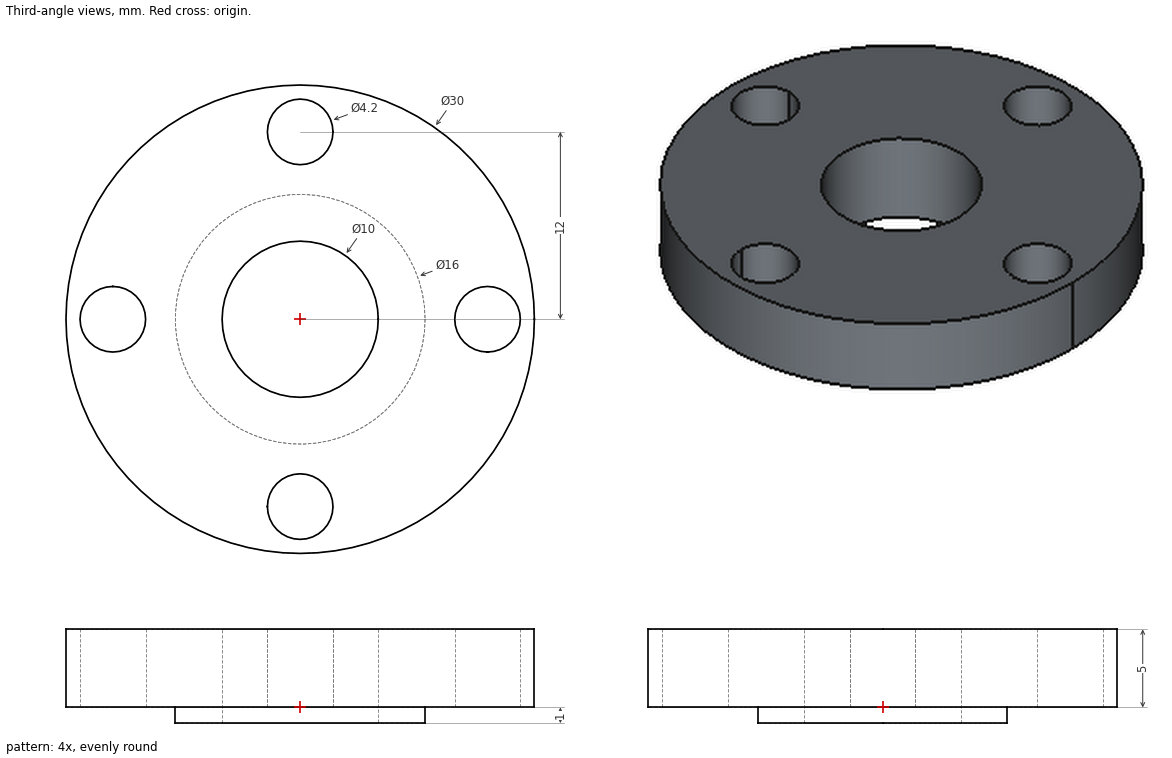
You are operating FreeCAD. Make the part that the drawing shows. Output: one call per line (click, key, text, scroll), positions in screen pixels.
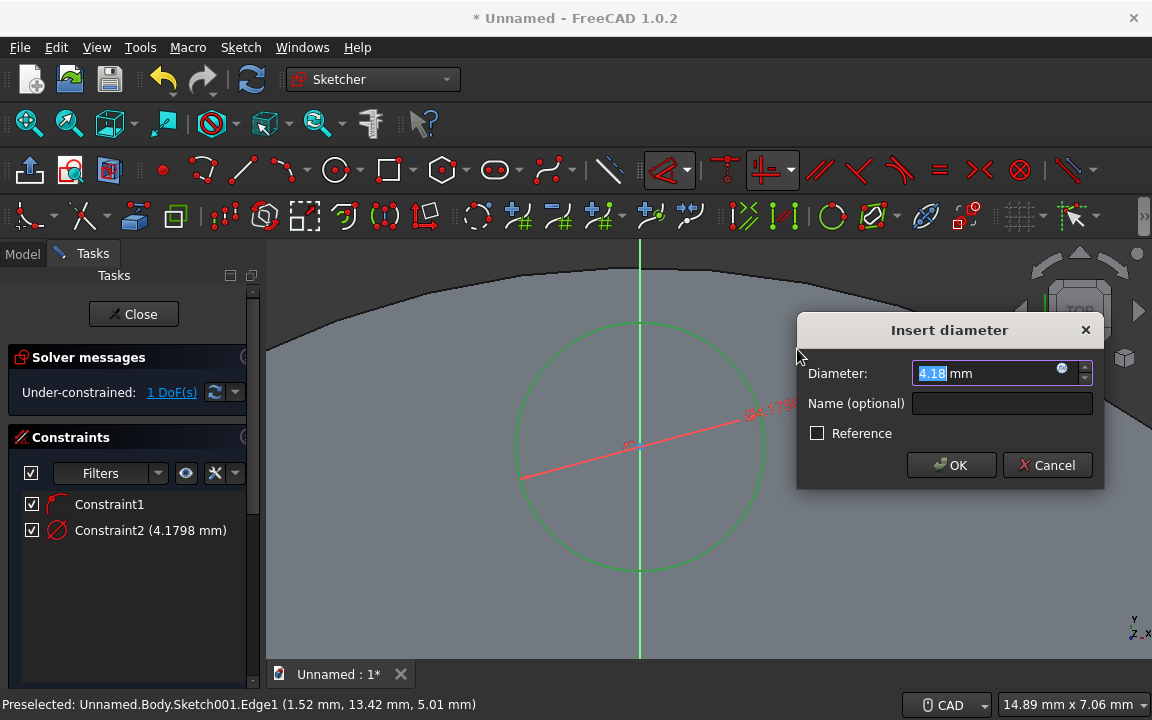
text(4.2)
key(Return)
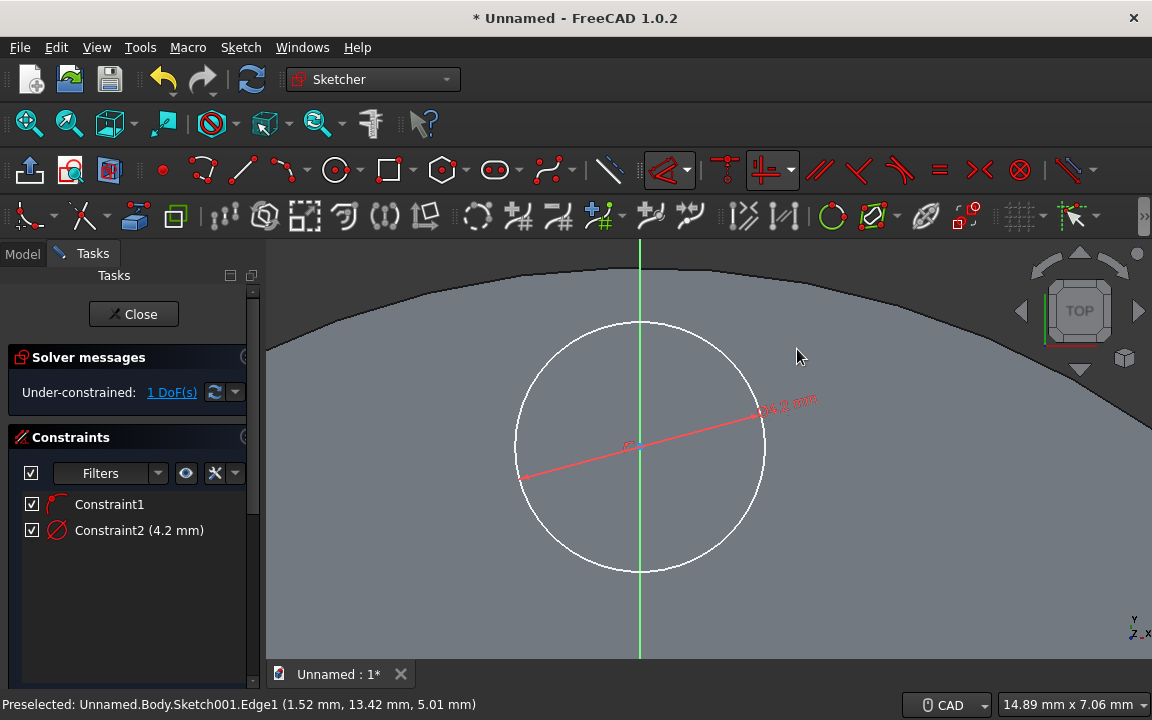
click(640, 447)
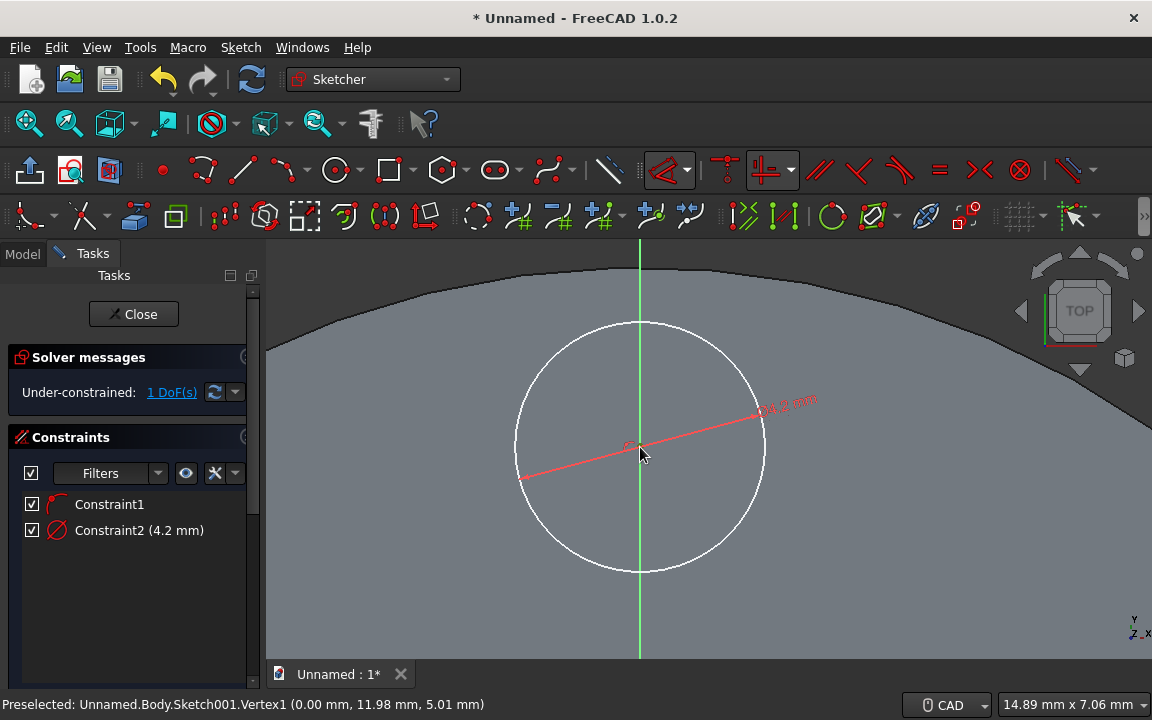
key(i)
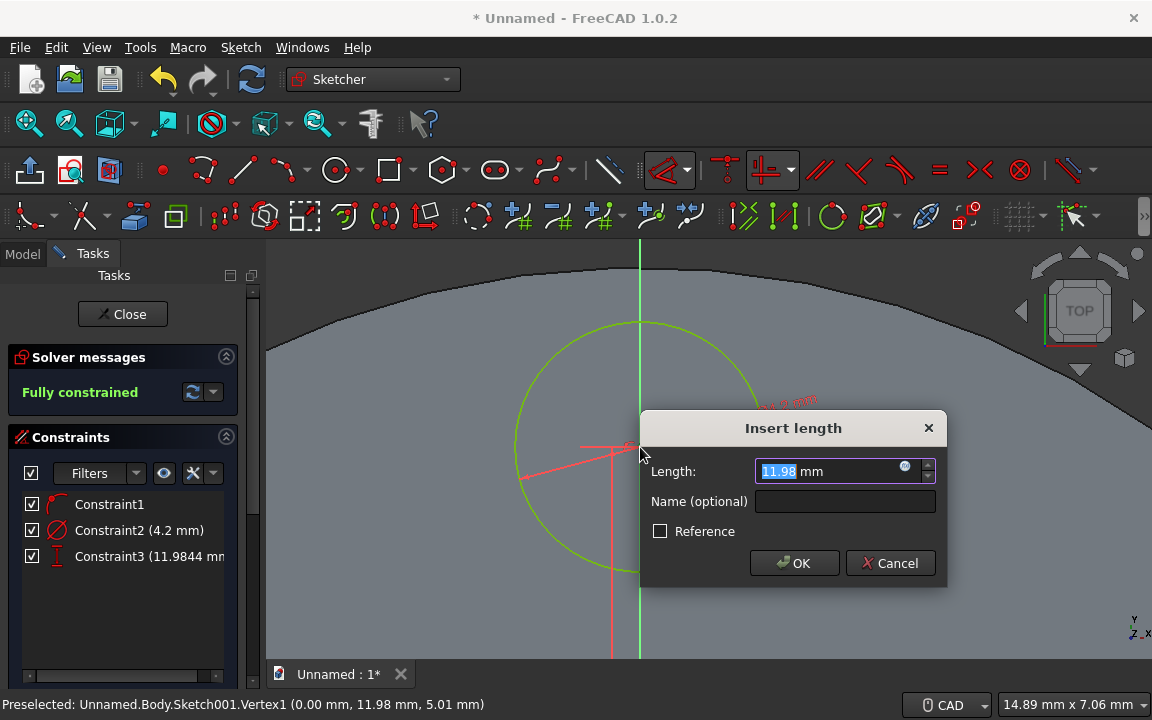
text(12)
key(Return)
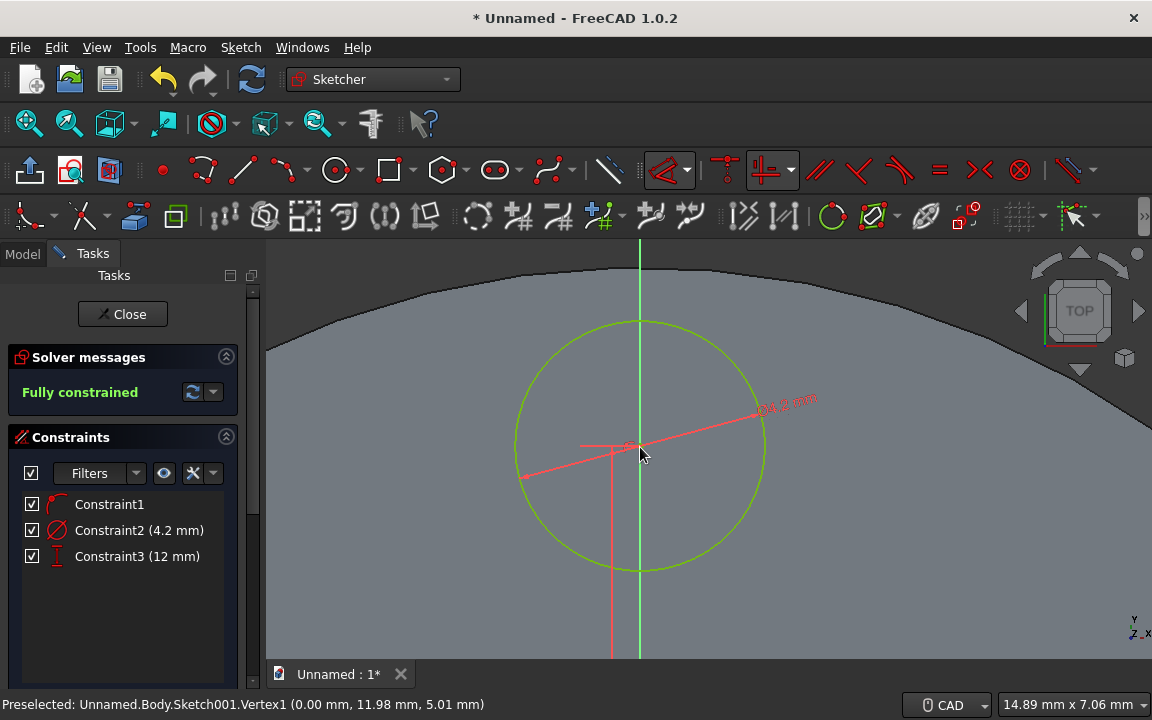
click(123, 314)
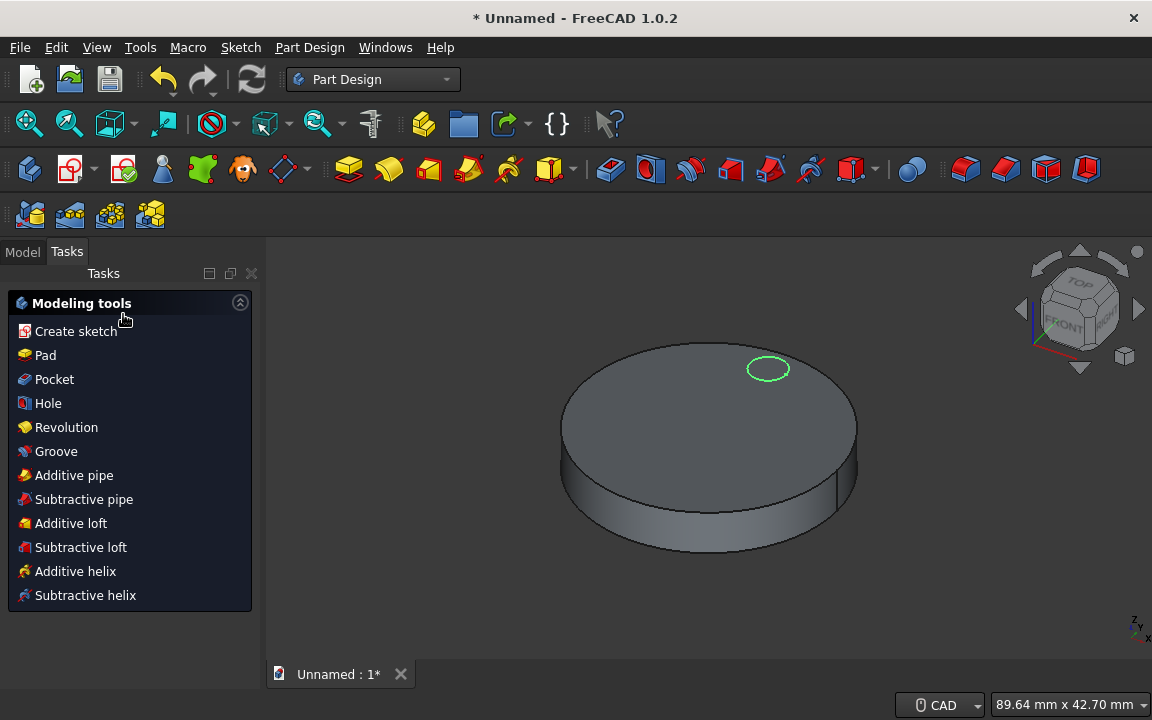
click(612, 170)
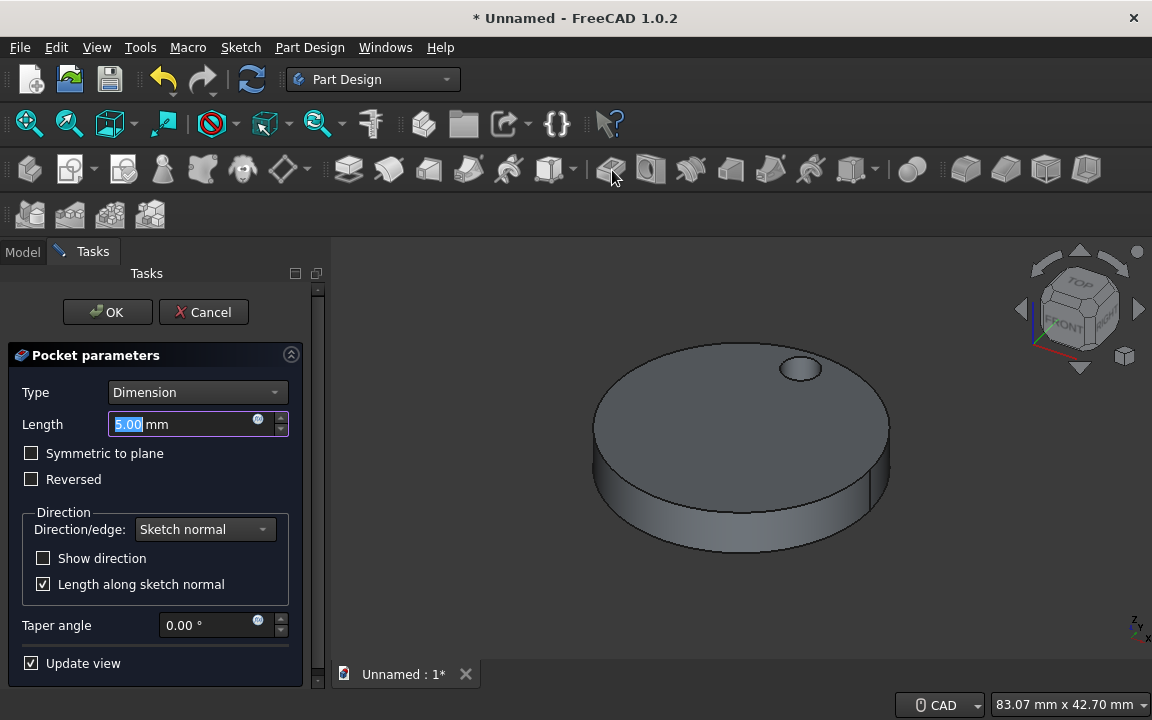
click(198, 392)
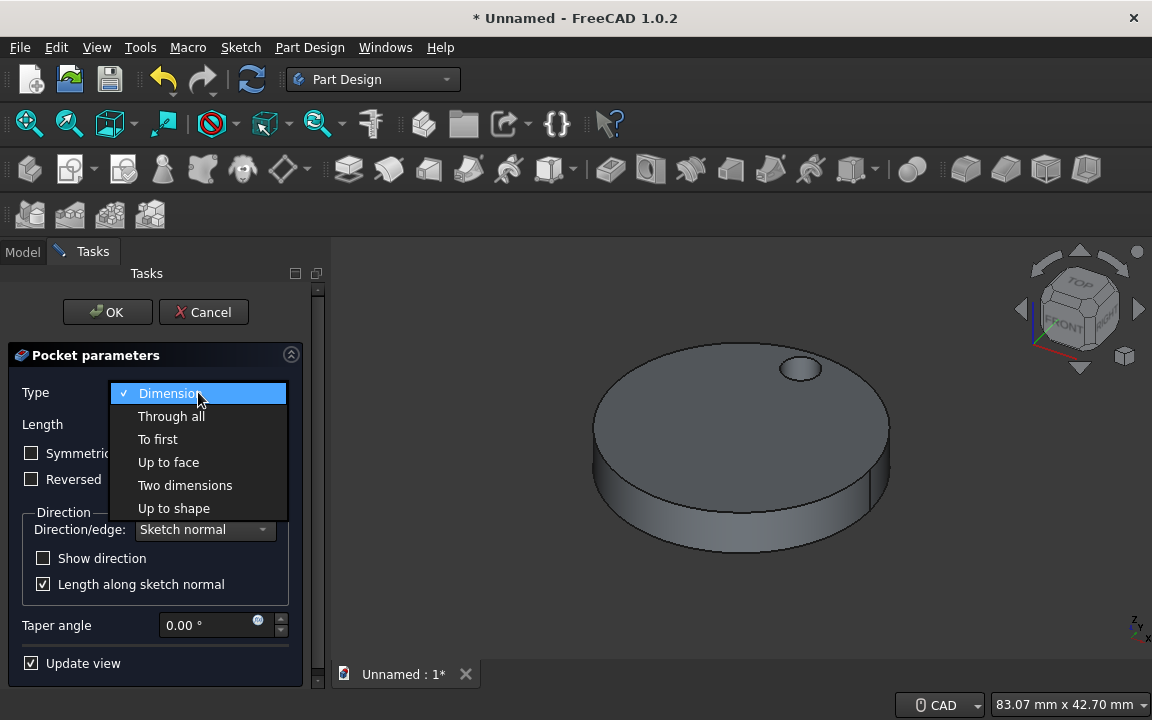
click(198, 416)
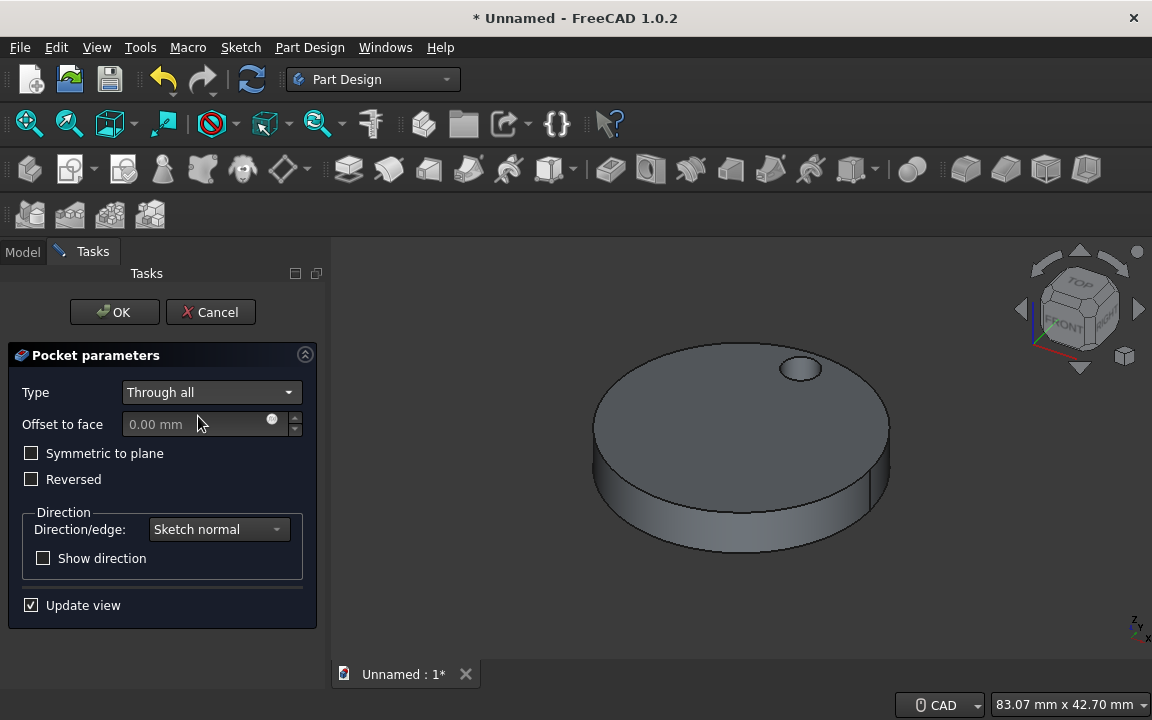
click(115, 312)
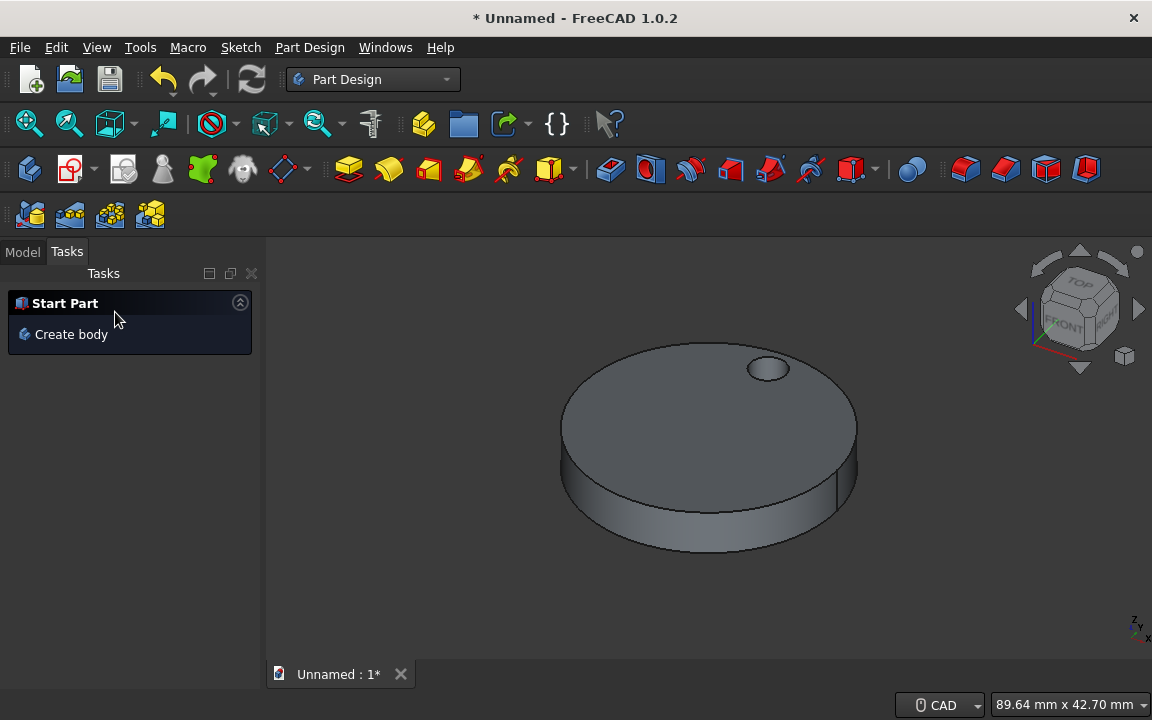
click(23, 251)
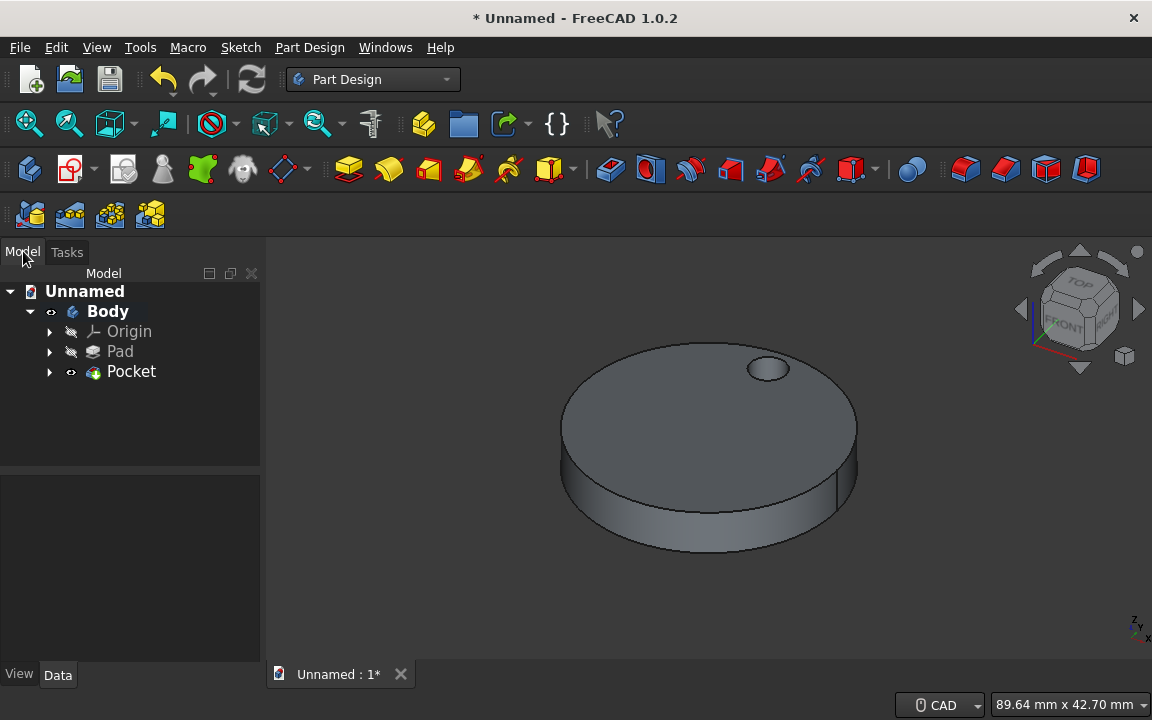
click(116, 372)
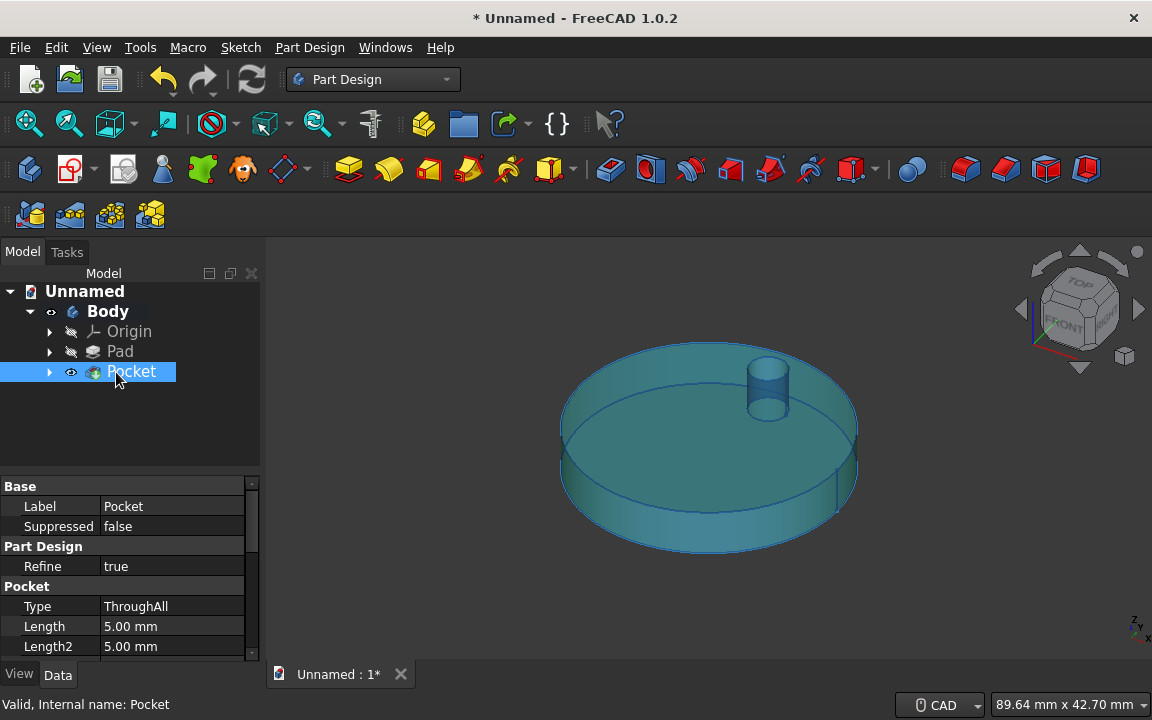
click(110, 214)